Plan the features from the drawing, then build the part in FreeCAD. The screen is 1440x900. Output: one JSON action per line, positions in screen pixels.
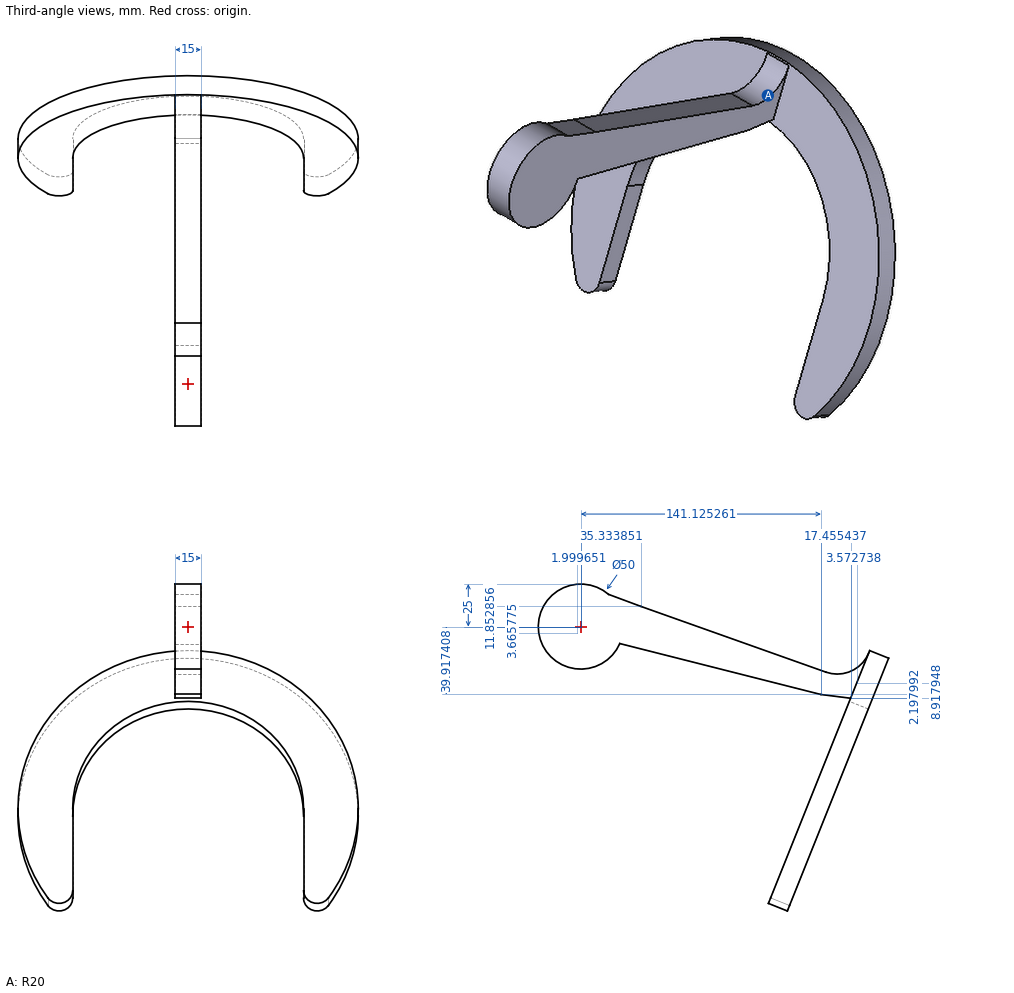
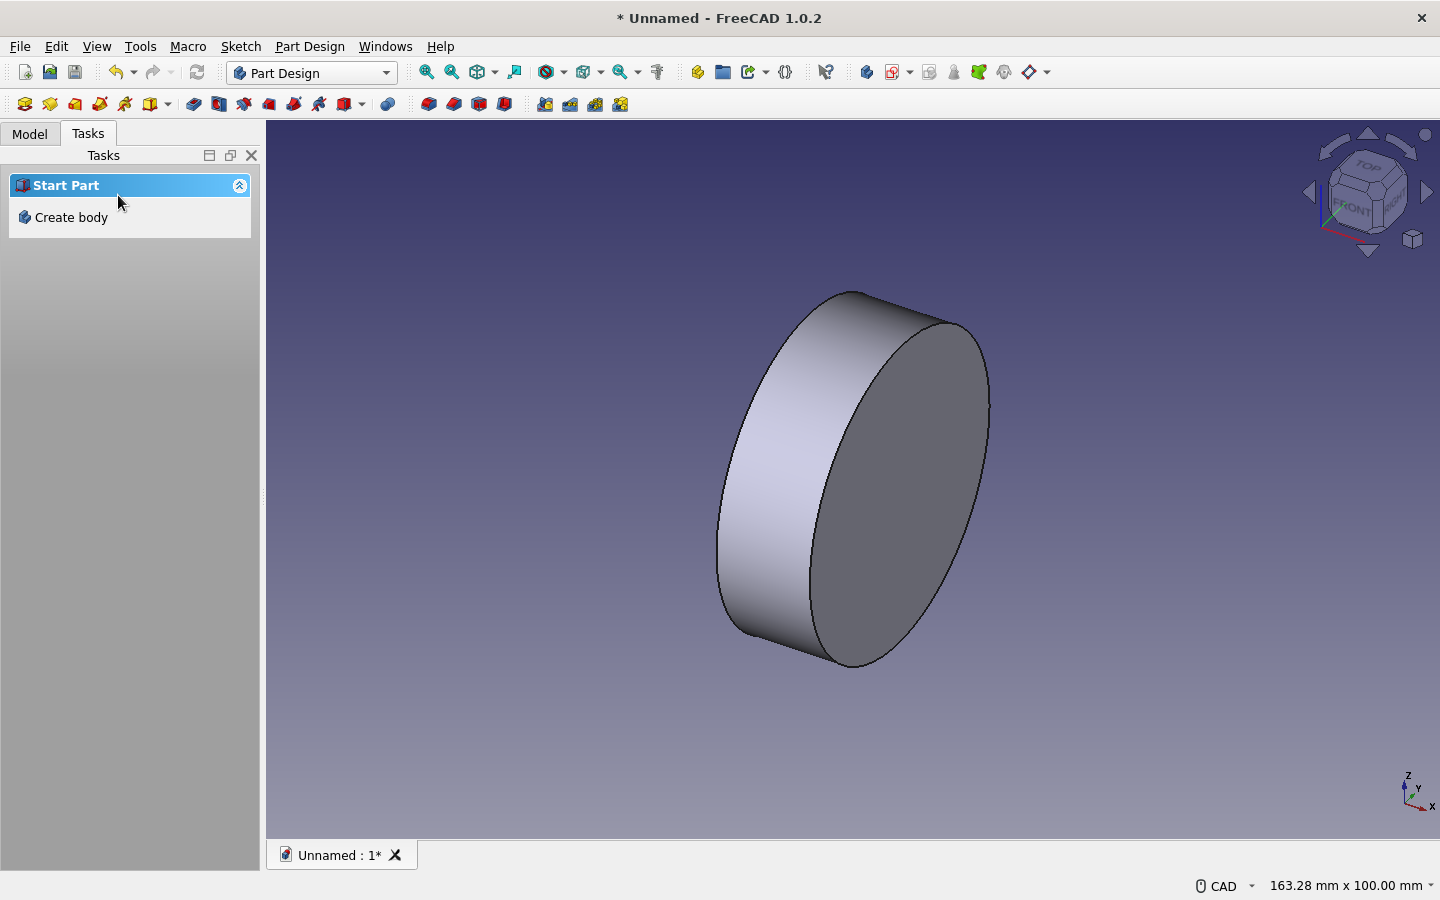
{"action": "left_click", "coordinate": [892, 72]}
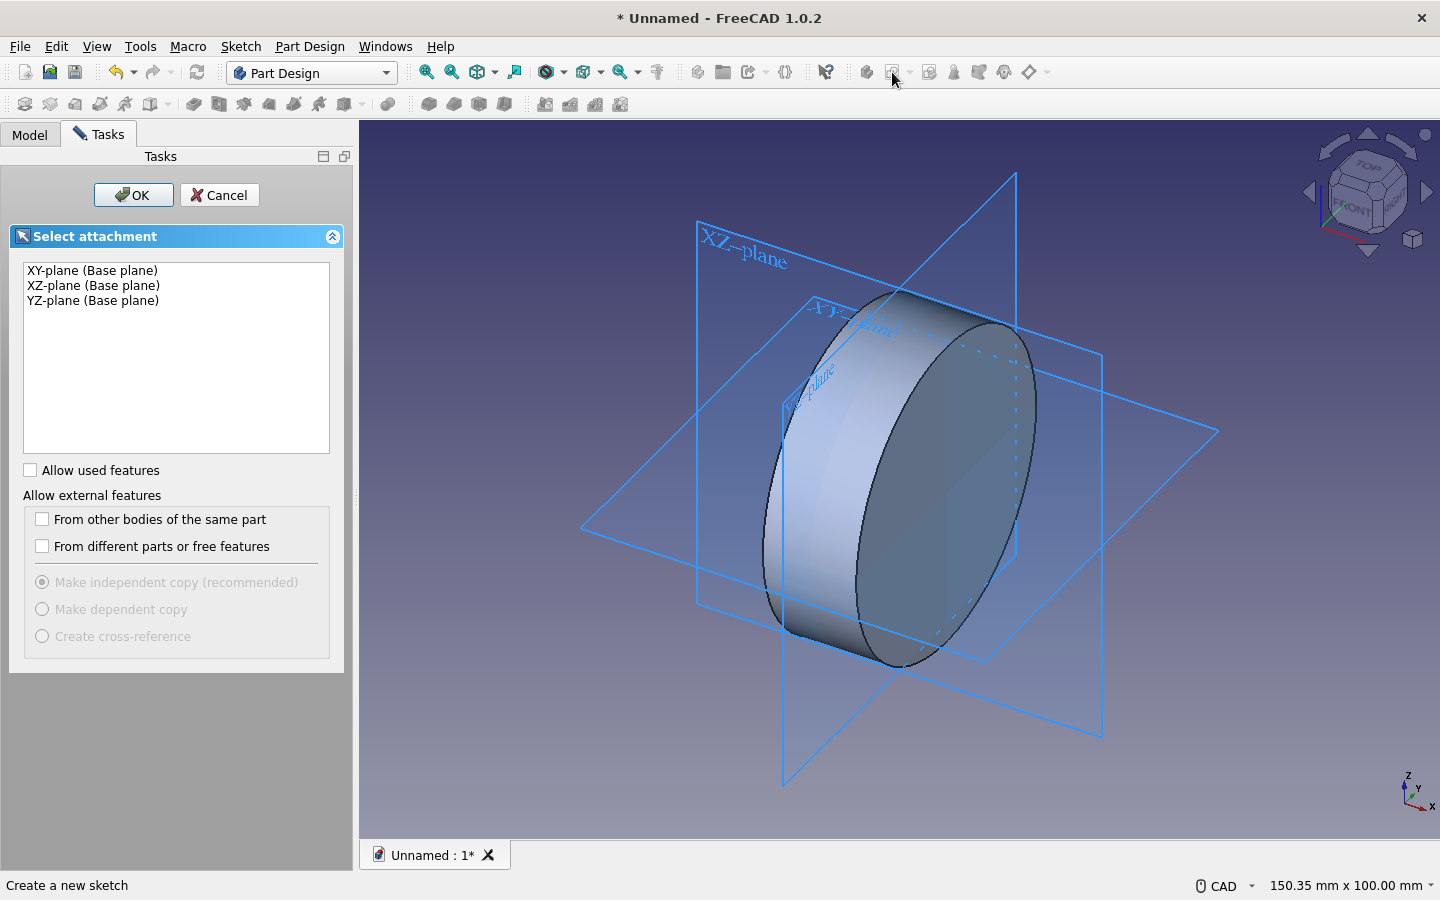
{"action": "left_click", "coordinate": [84, 300]}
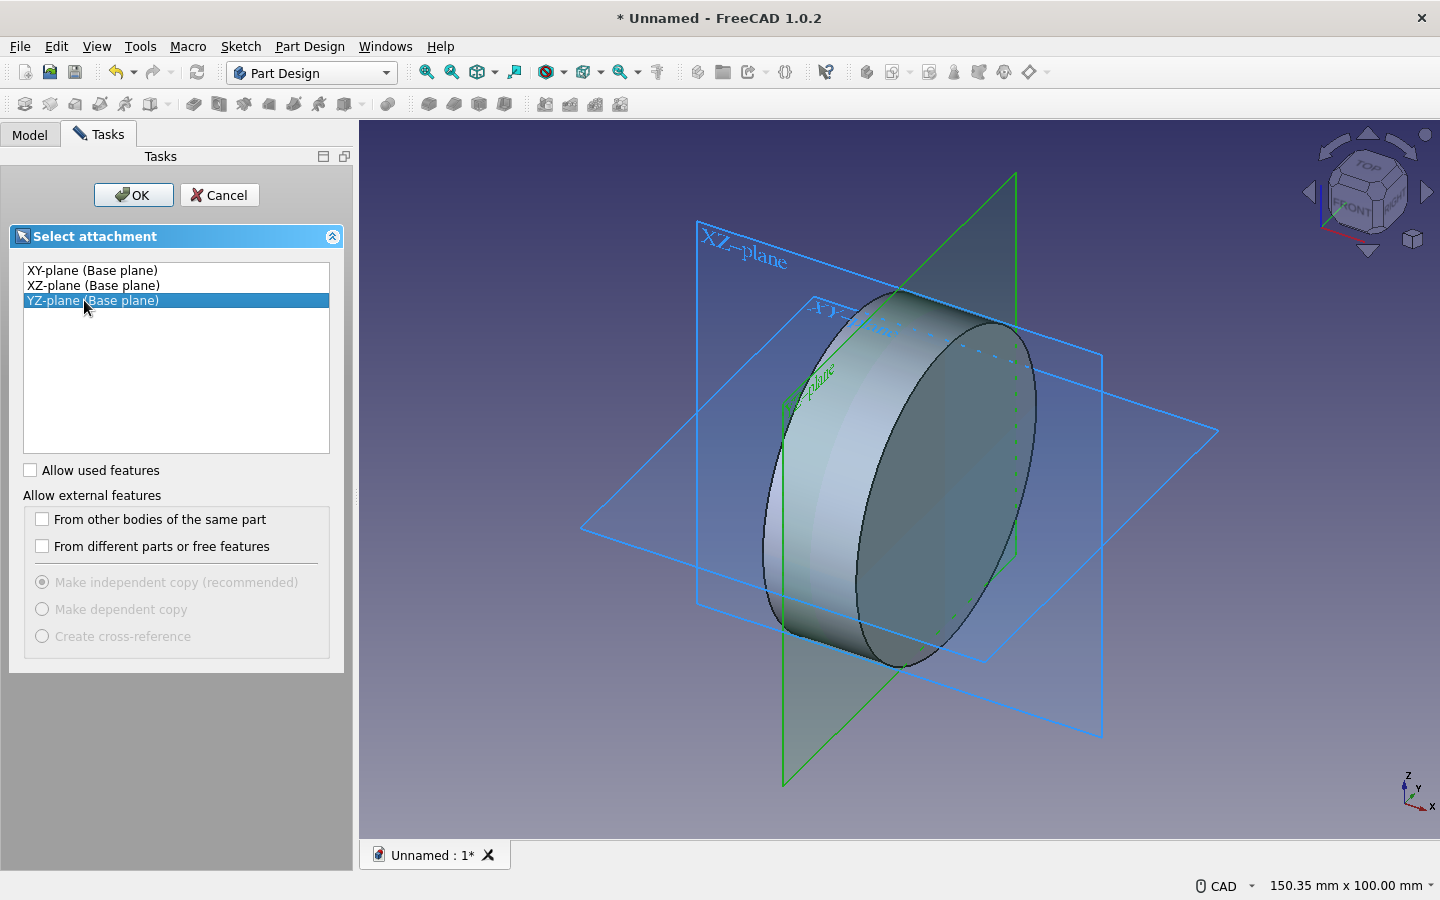
{"action": "left_click", "coordinate": [134, 195]}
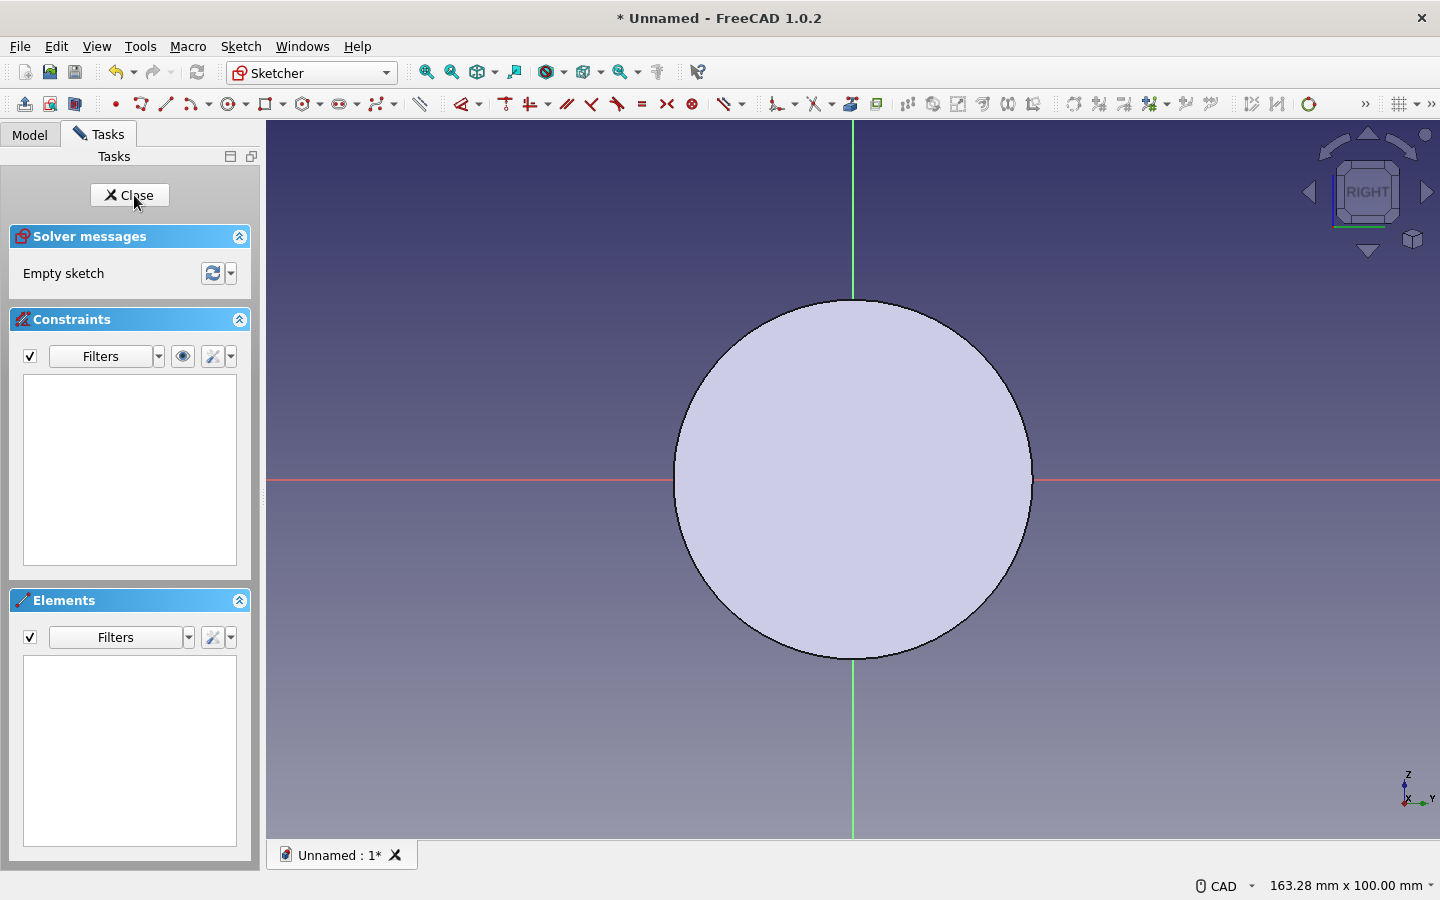
{"action": "key", "text": "q s"}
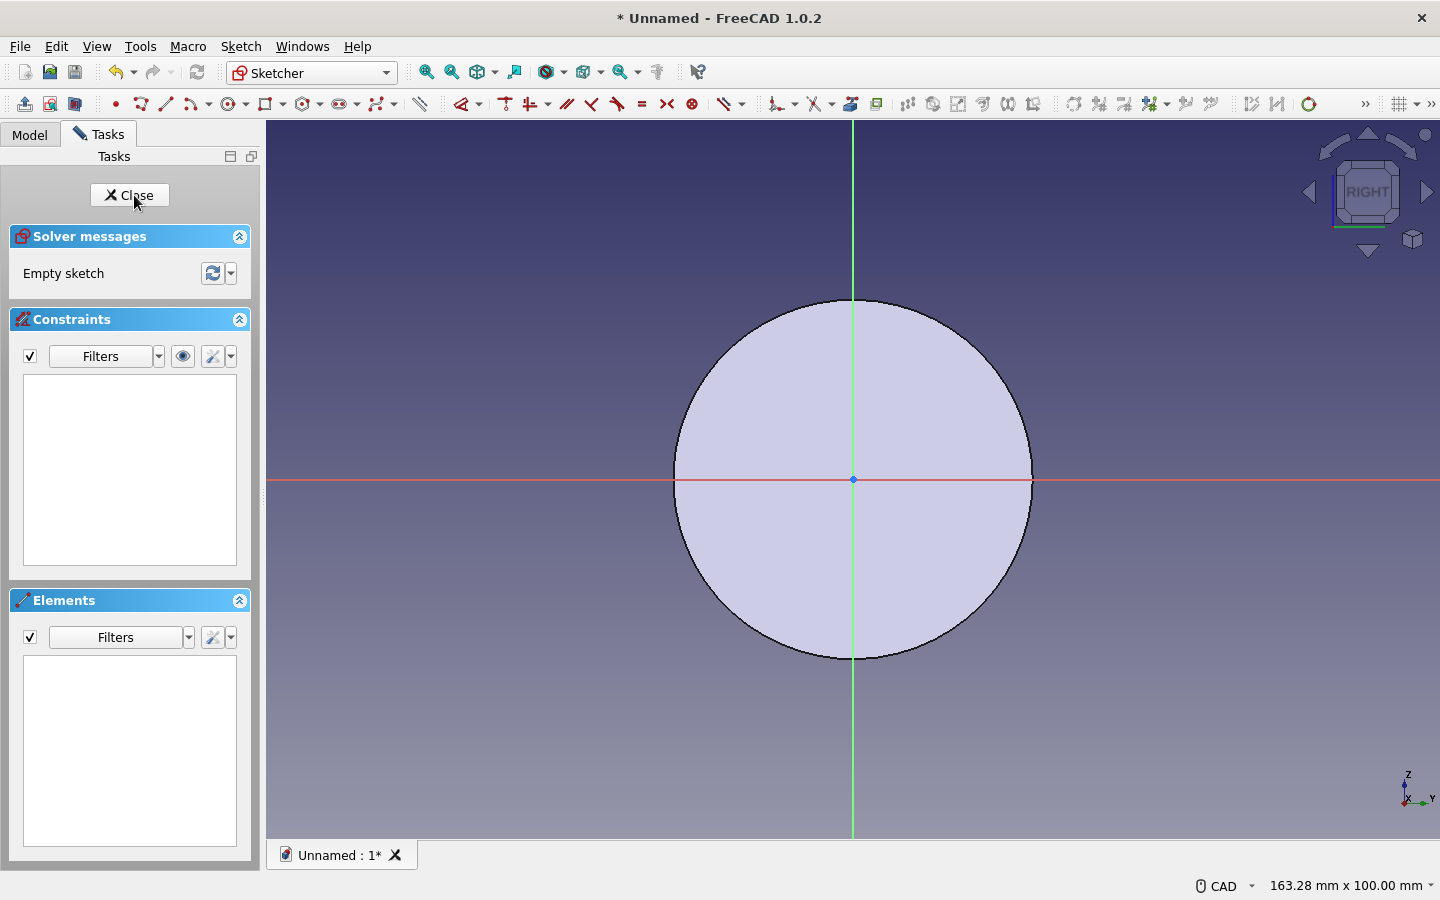
{"action": "scroll", "coordinate": [294, 405], "scroll_direction": "down", "scroll_amount": 3}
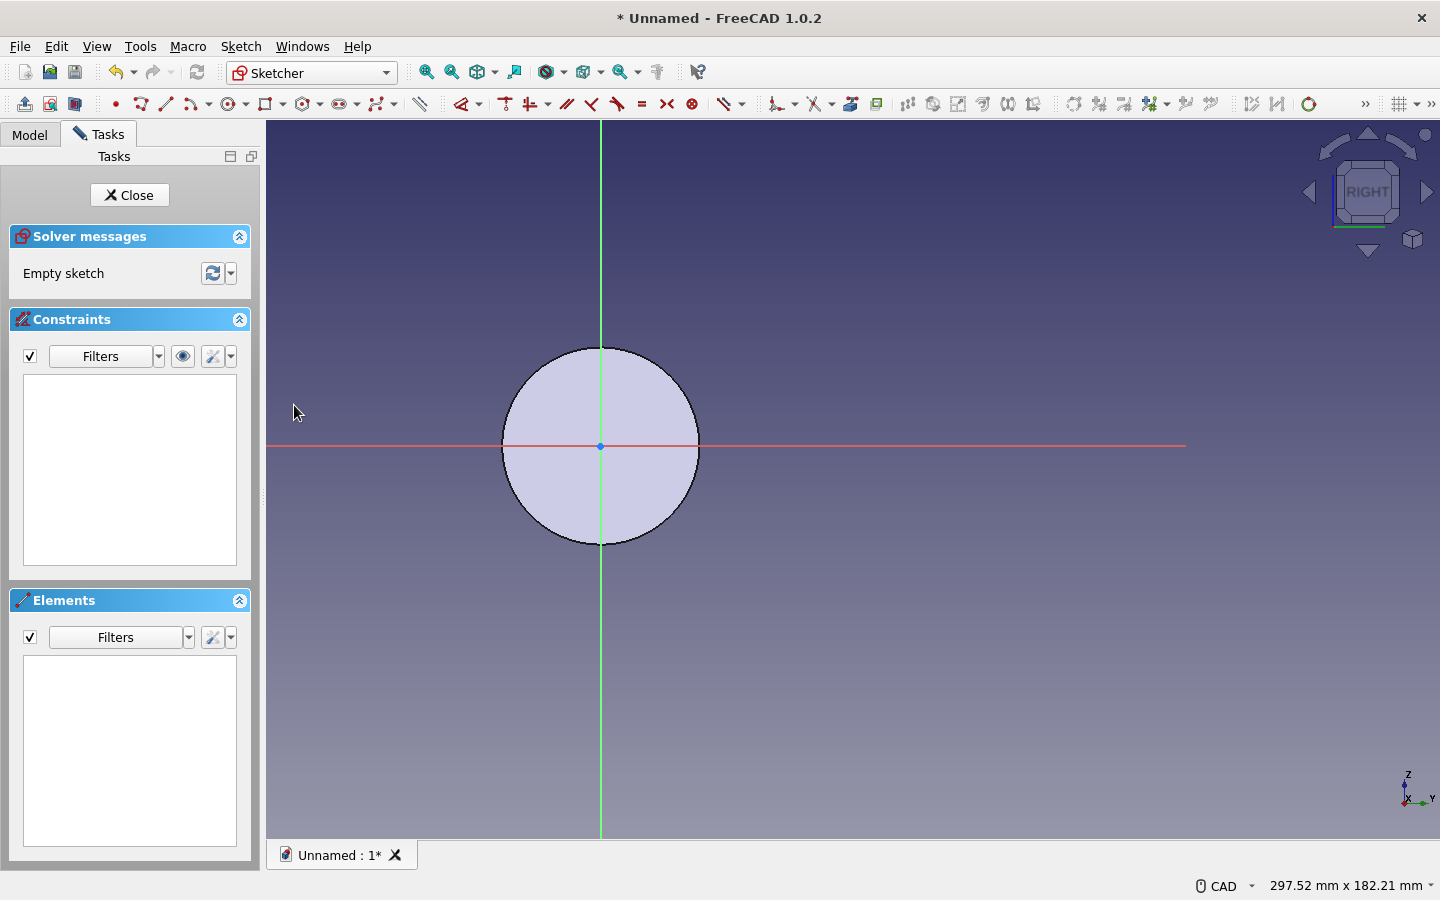
{"action": "left_click", "coordinate": [141, 104]}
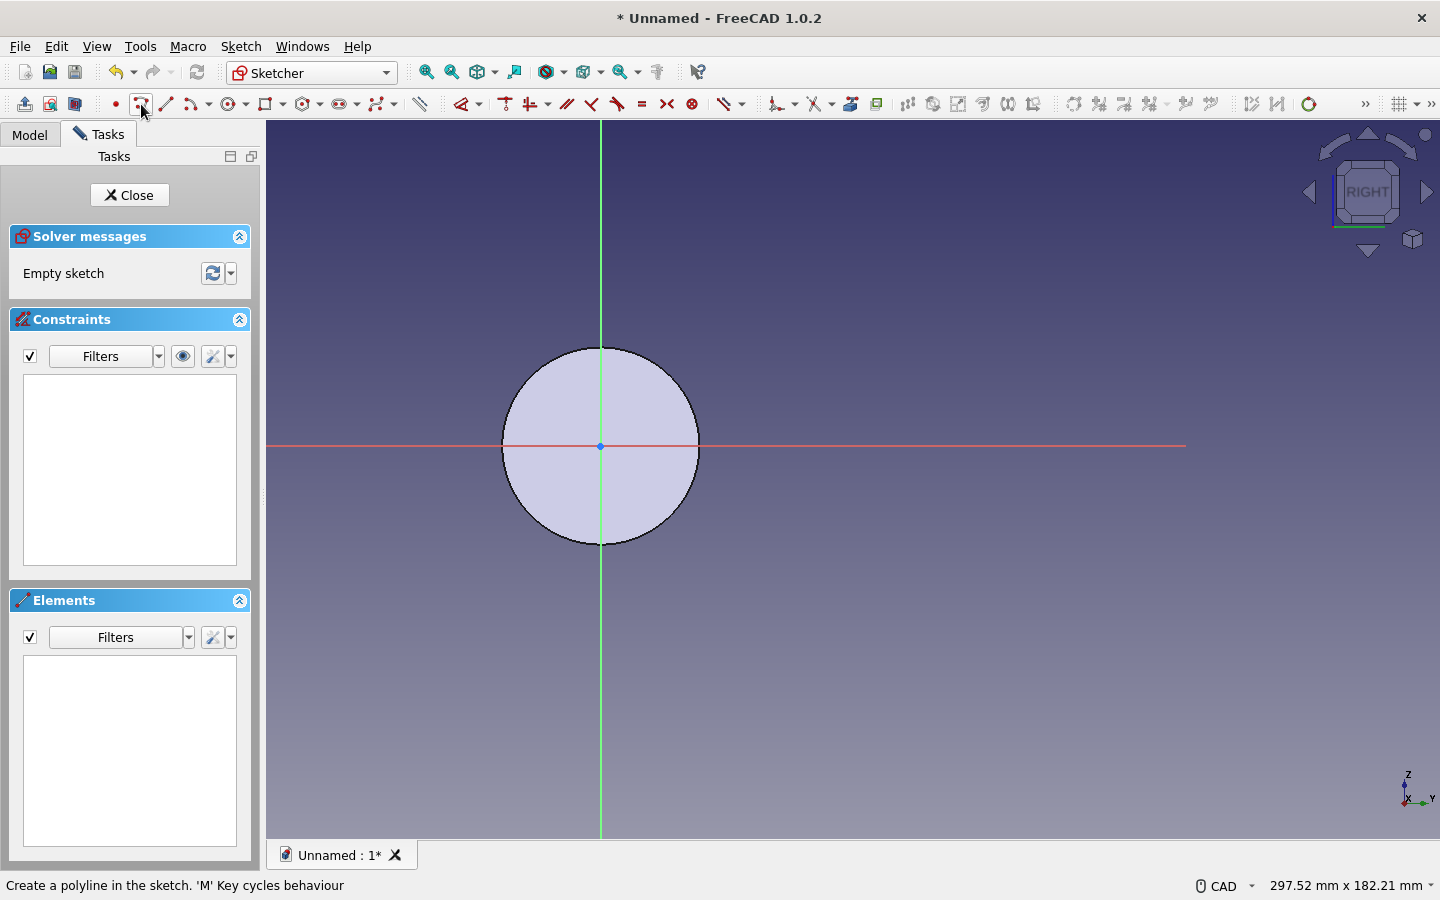
{"action": "scroll", "coordinate": [593, 461], "scroll_direction": "up", "scroll_amount": 4}